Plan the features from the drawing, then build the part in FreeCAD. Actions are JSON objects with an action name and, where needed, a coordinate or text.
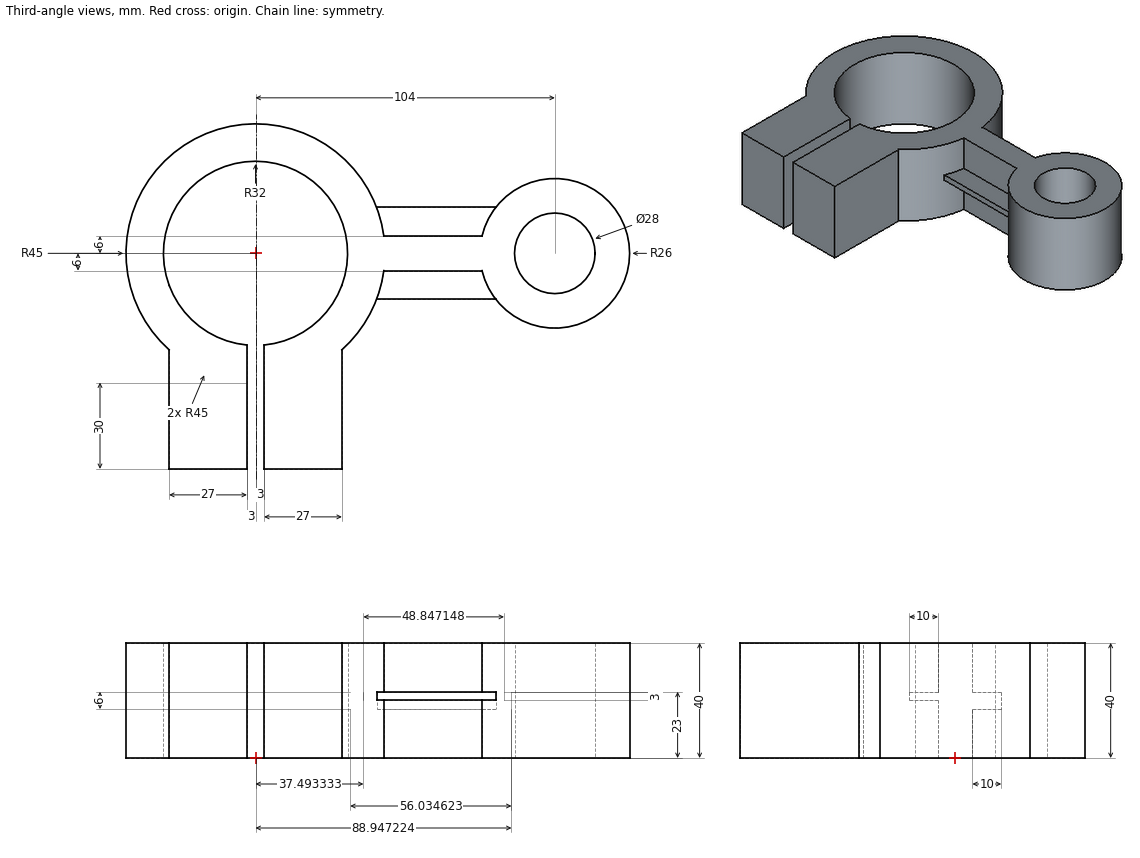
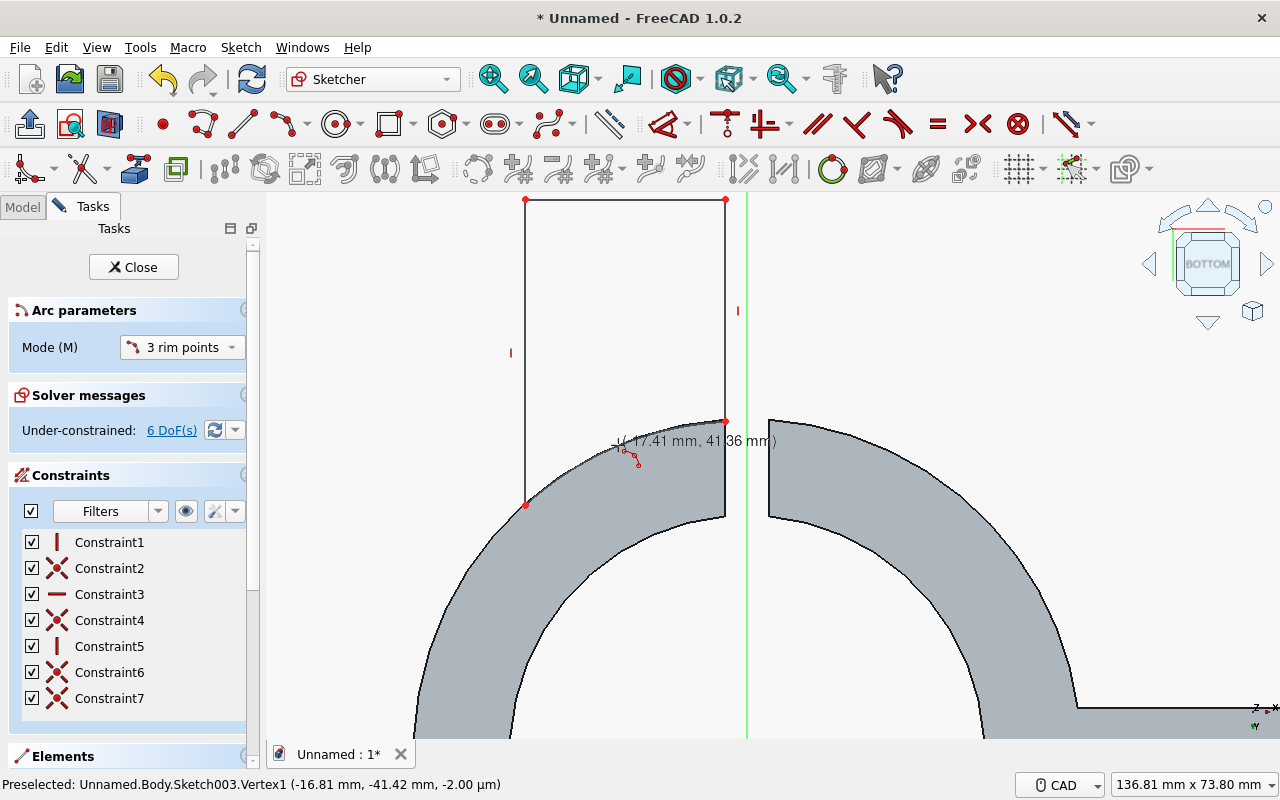
{"action": "key", "text": "g m"}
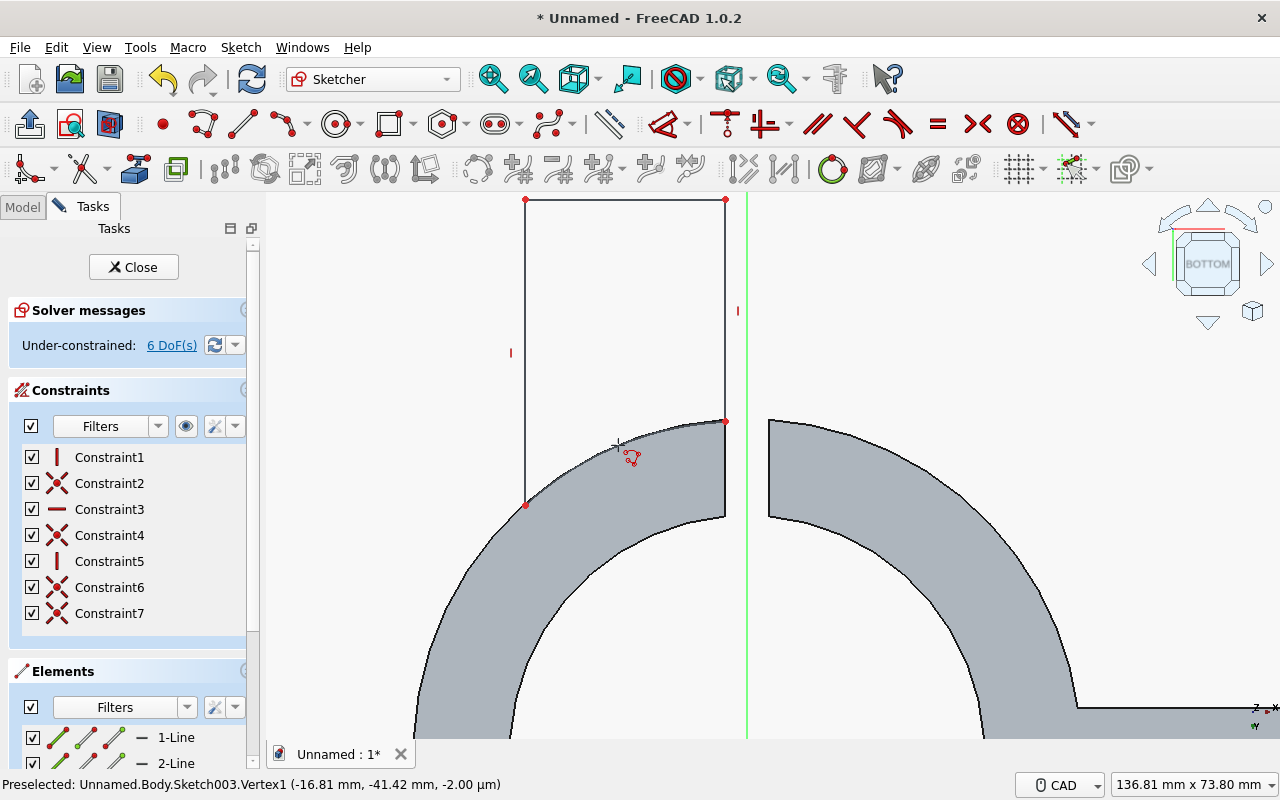
{"action": "left_click", "coordinate": [769, 420]}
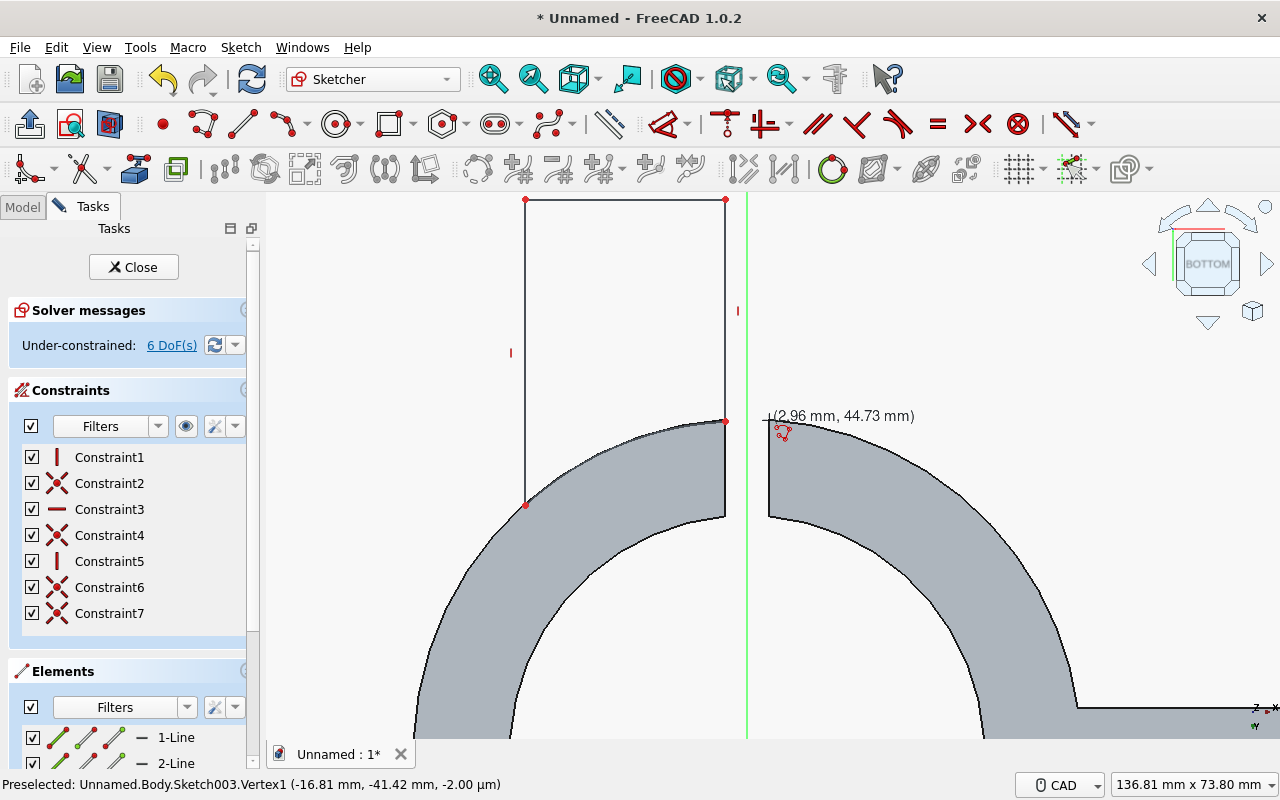
{"action": "scroll", "coordinate": [618, 446], "scroll_direction": "down", "scroll_amount": 2}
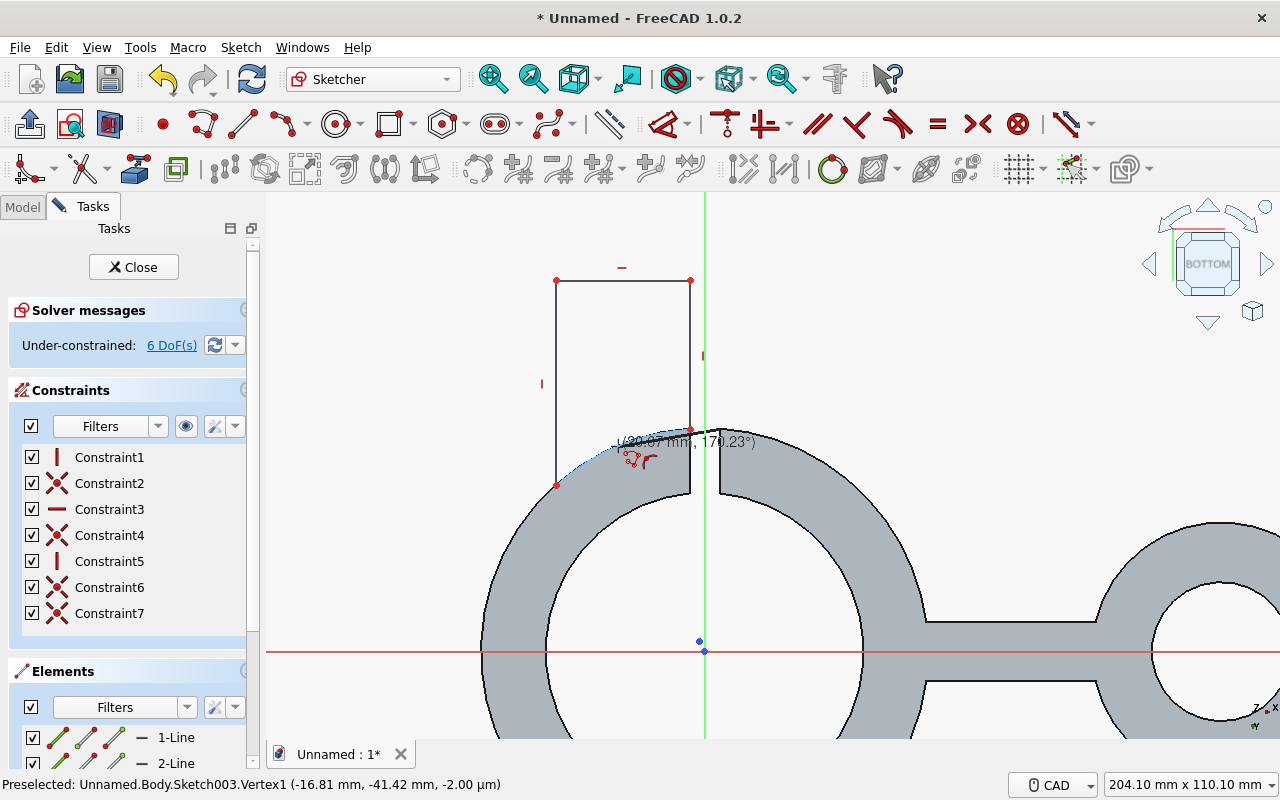
{"action": "left_click", "coordinate": [719, 280]}
{"action": "left_click", "coordinate": [854, 280]}
{"action": "left_click", "coordinate": [854, 485]}
{"action": "right_click", "coordinate": [854, 485]}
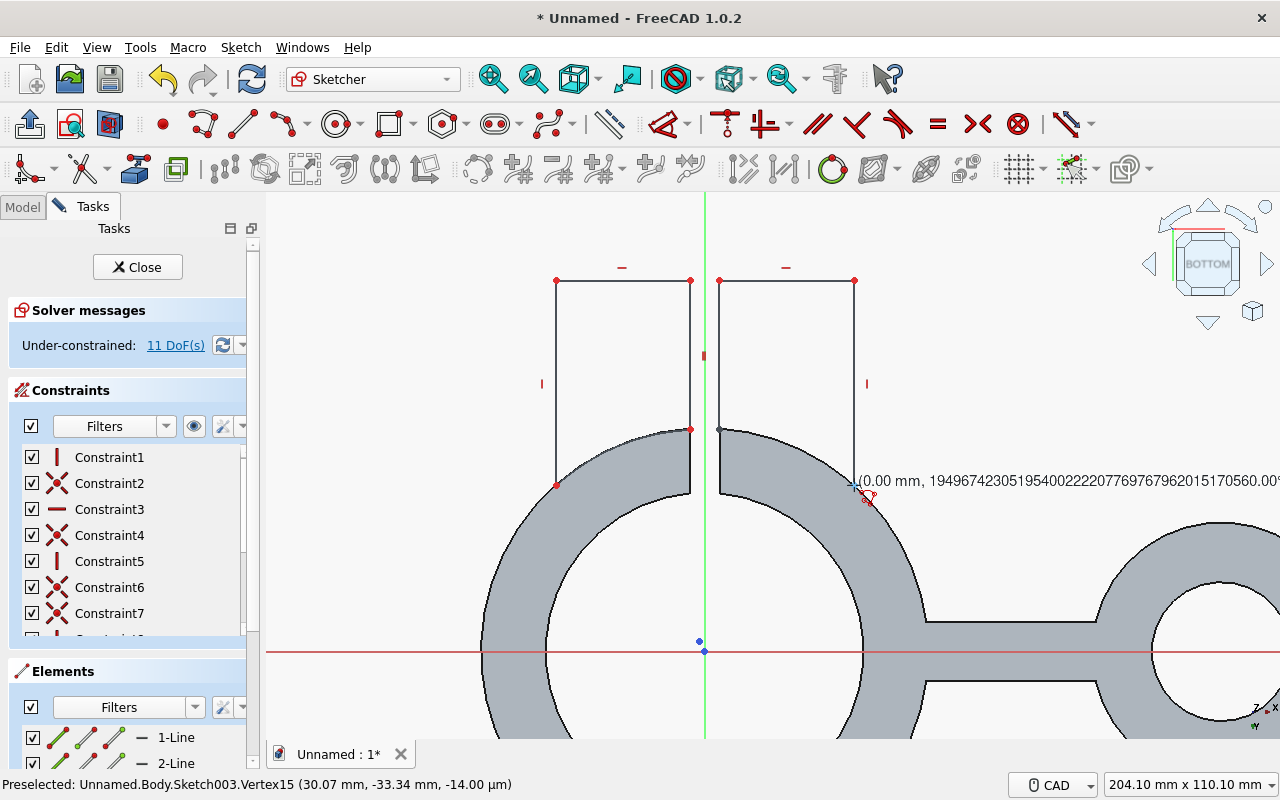
{"action": "key", "text": "g 3 a"}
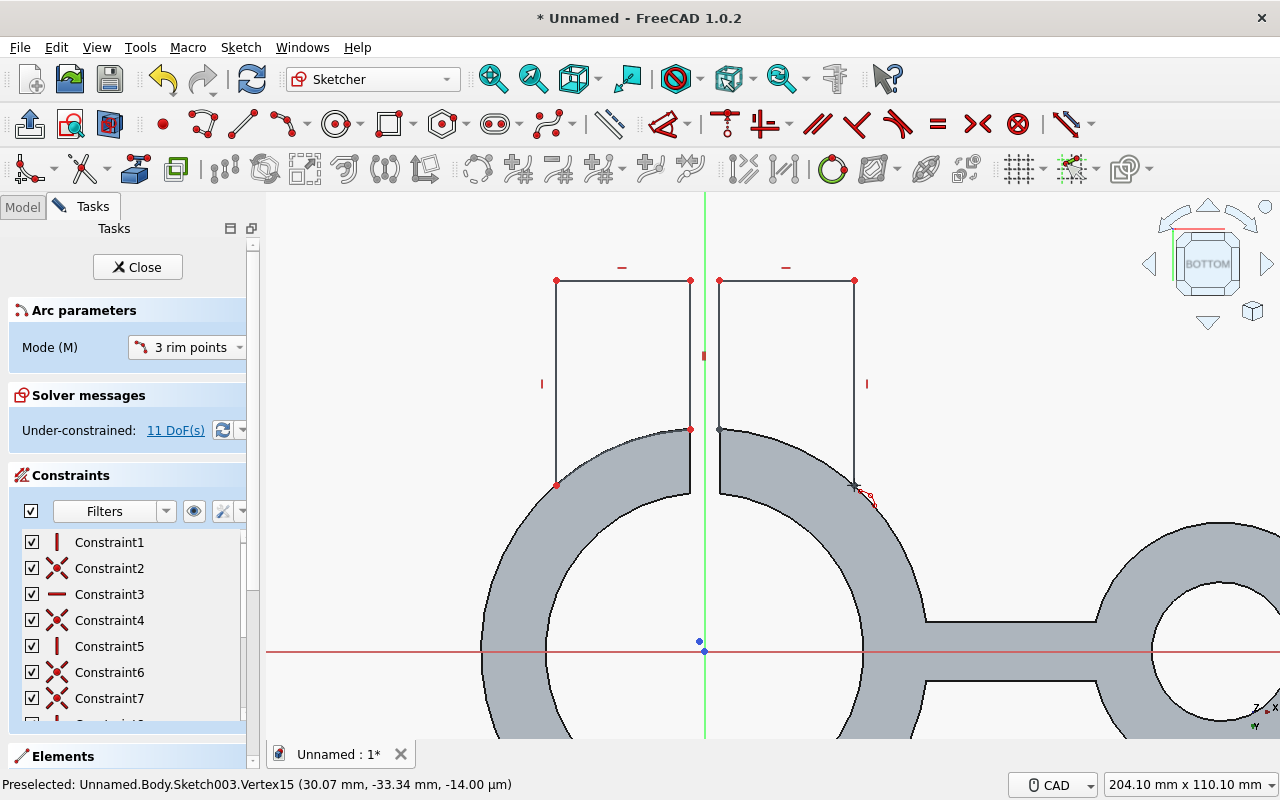
{"action": "left_click", "coordinate": [854, 486]}
{"action": "left_click", "coordinate": [719, 429]}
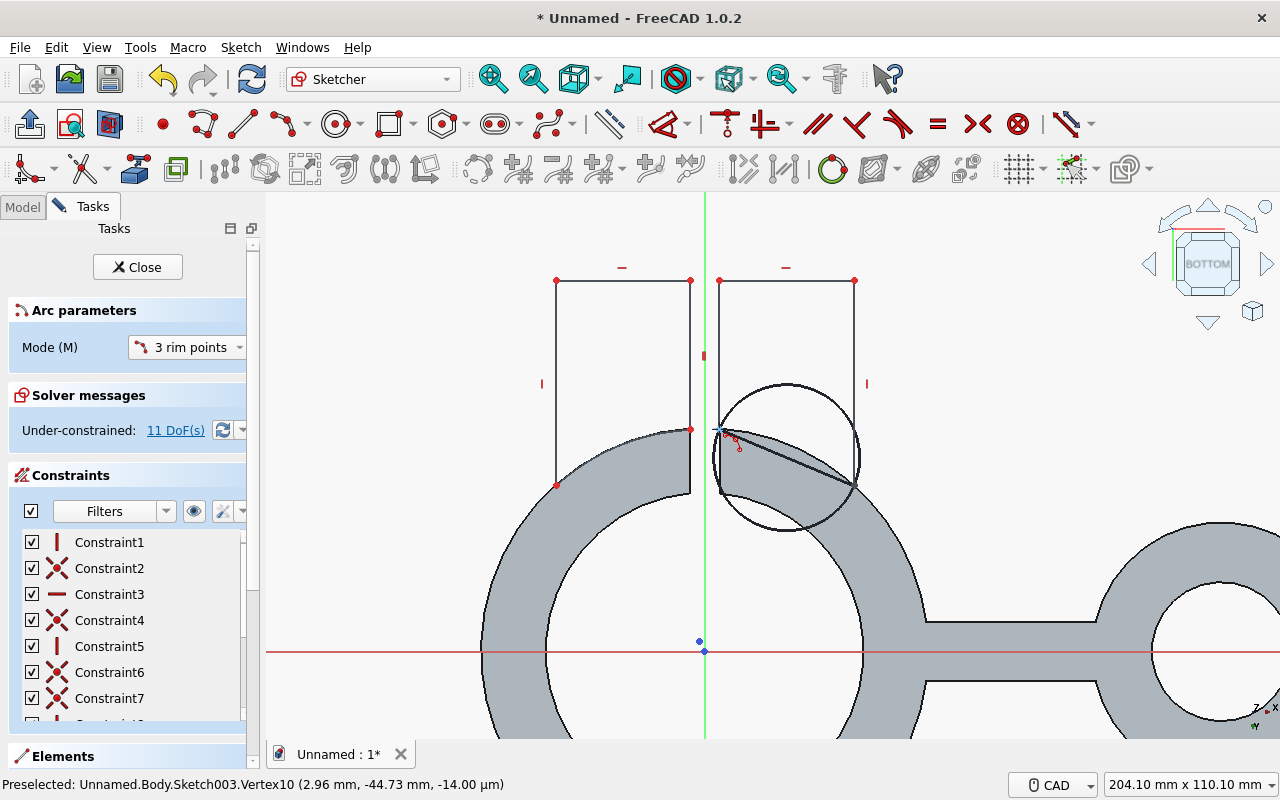
{"action": "scroll", "coordinate": [791, 446], "scroll_direction": "up", "scroll_amount": 2}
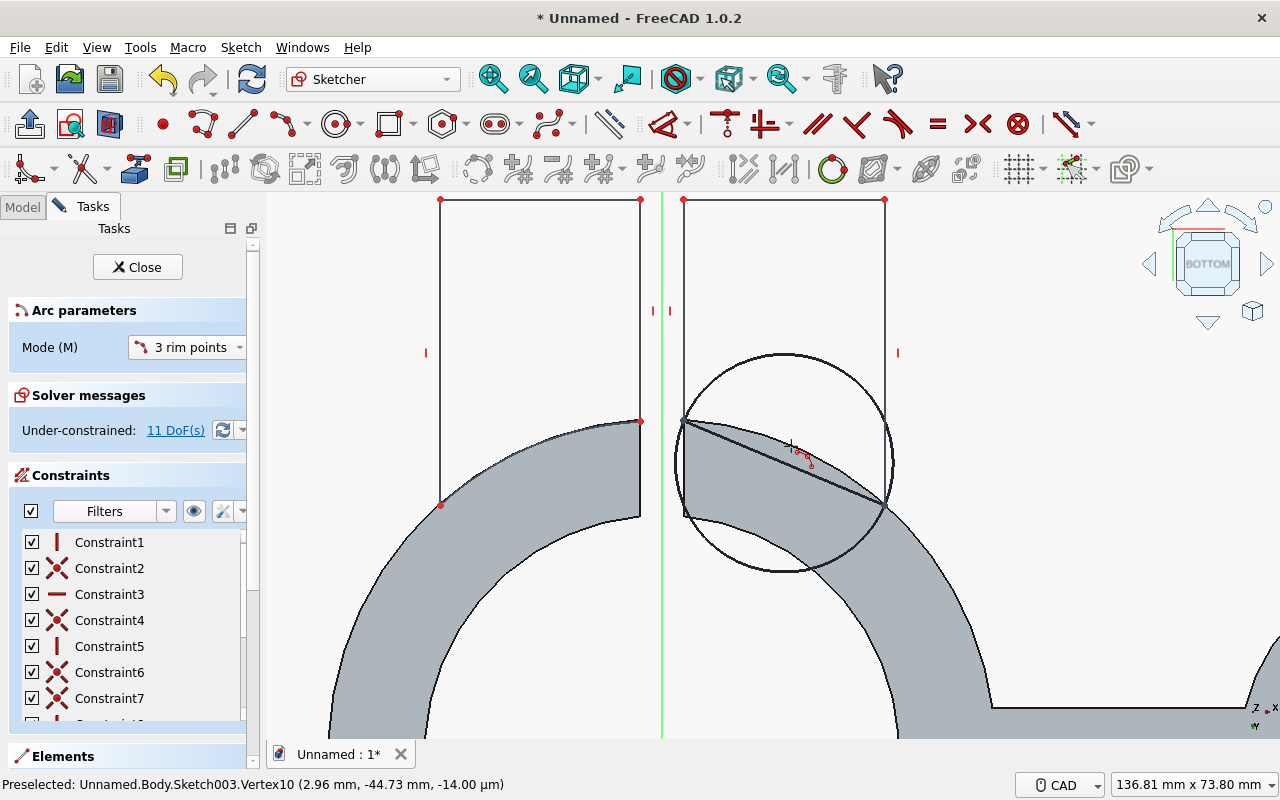
{"action": "left_click", "coordinate": [791, 445]}
{"action": "key", "text": "Escape"}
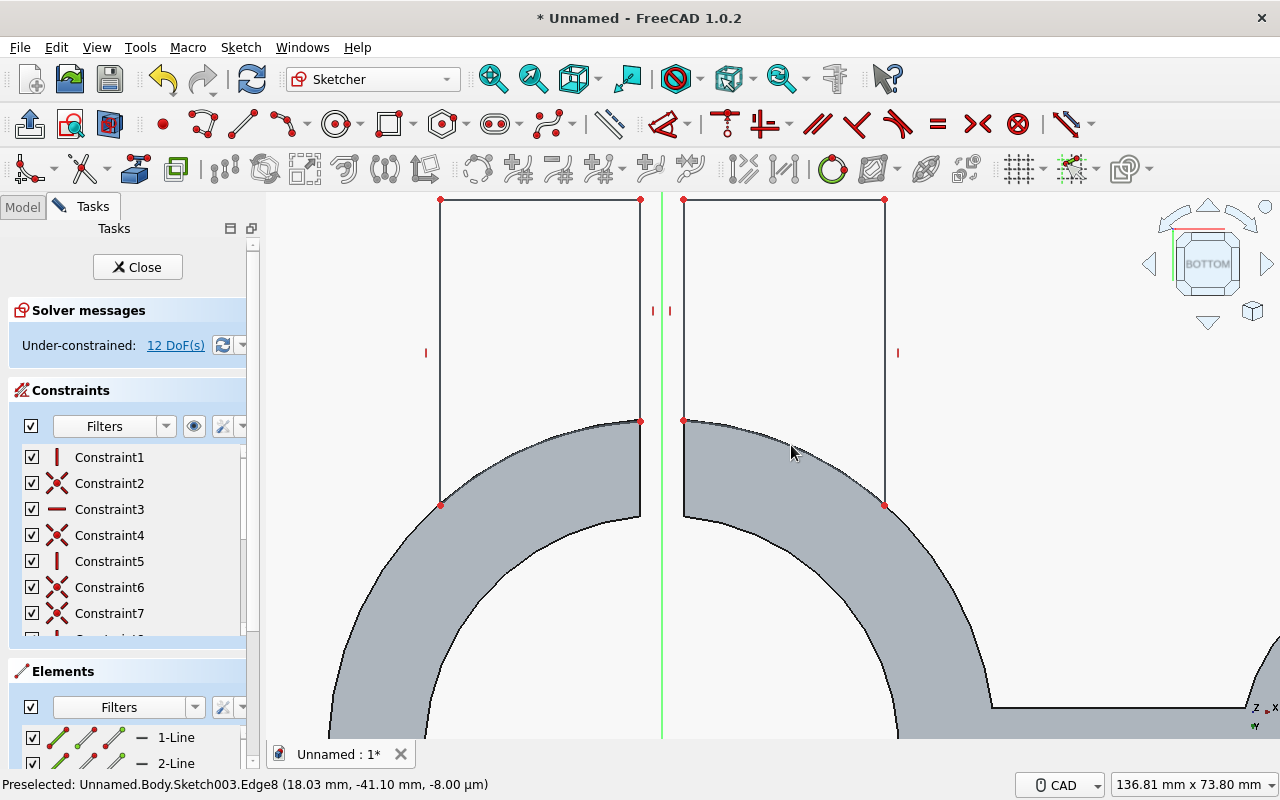
{"action": "left_click", "coordinate": [575, 432]}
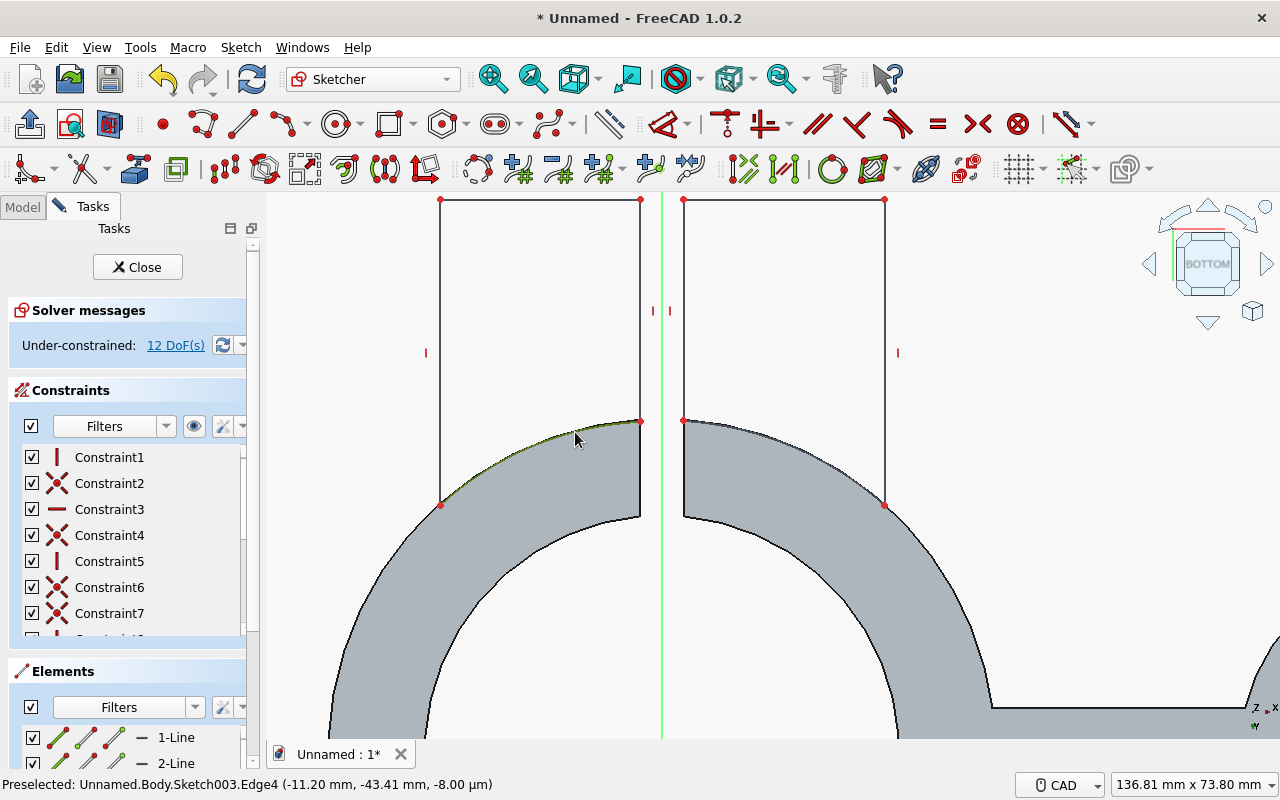
{"action": "left_click", "coordinate": [831, 466]}